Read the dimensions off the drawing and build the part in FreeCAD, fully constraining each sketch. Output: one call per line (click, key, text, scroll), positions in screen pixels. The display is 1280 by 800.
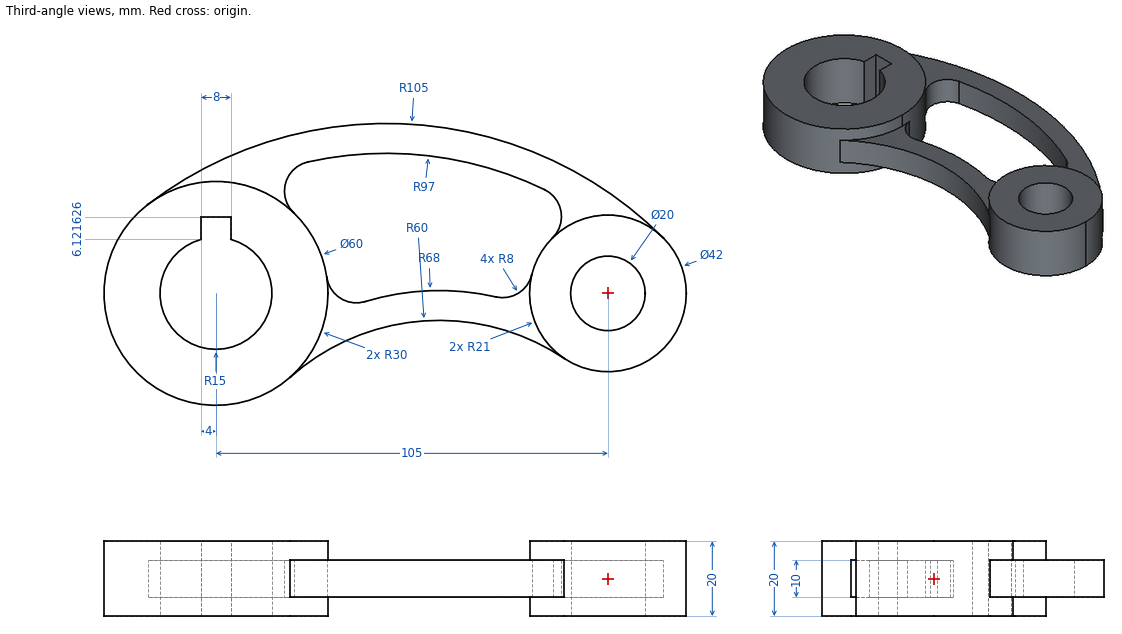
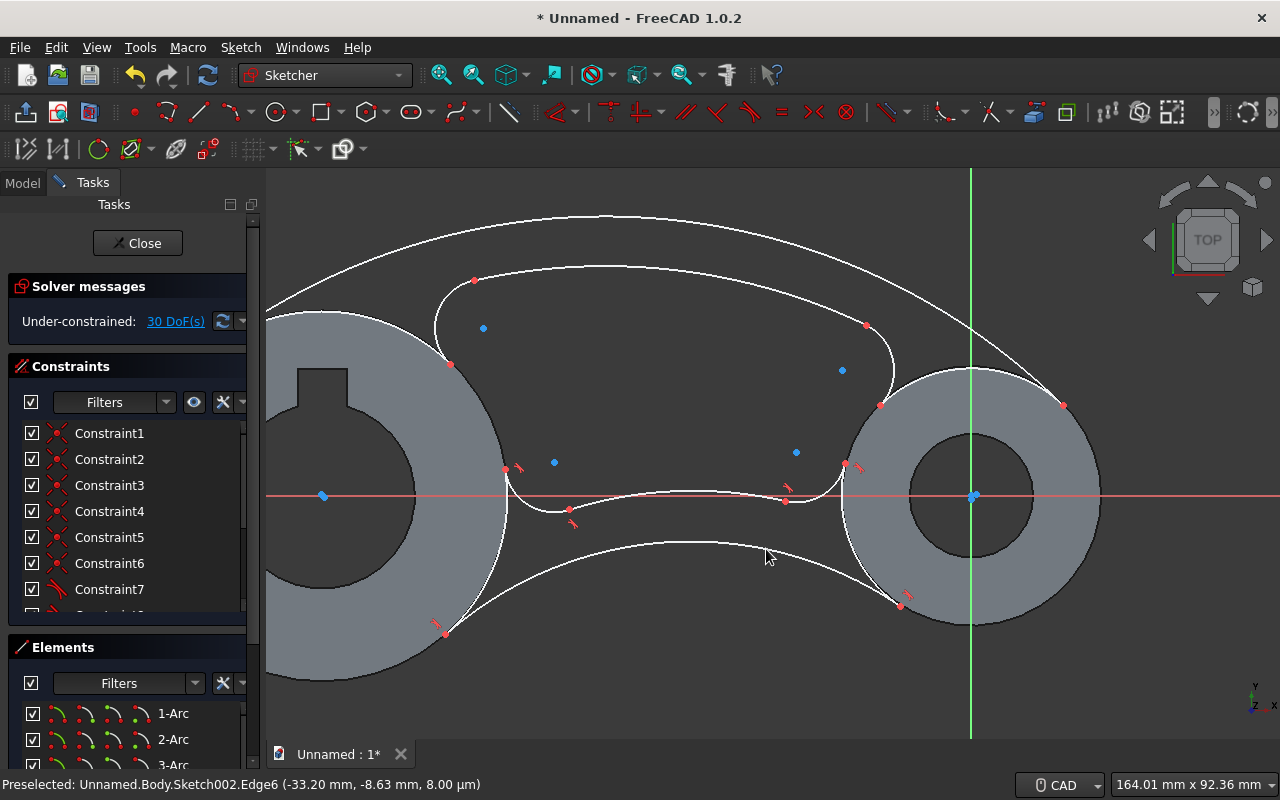
click(829, 256)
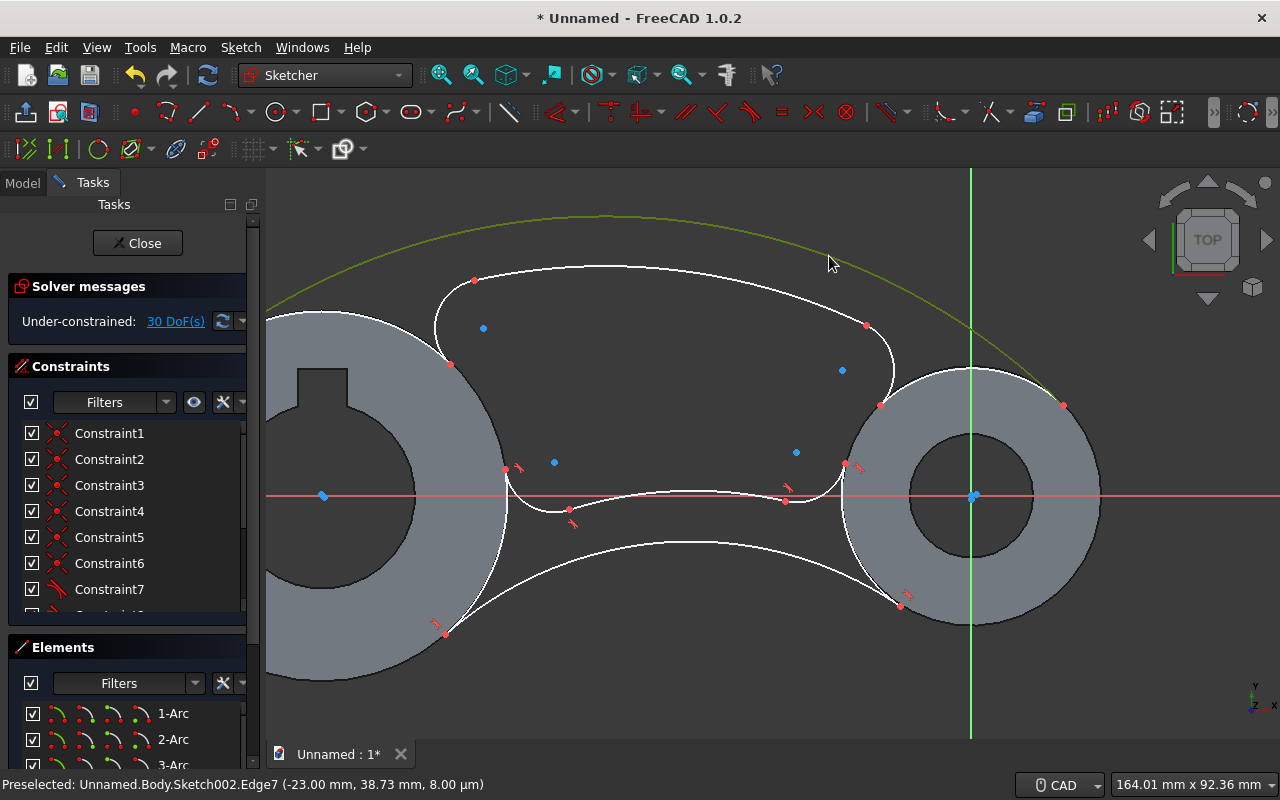
click(384, 322)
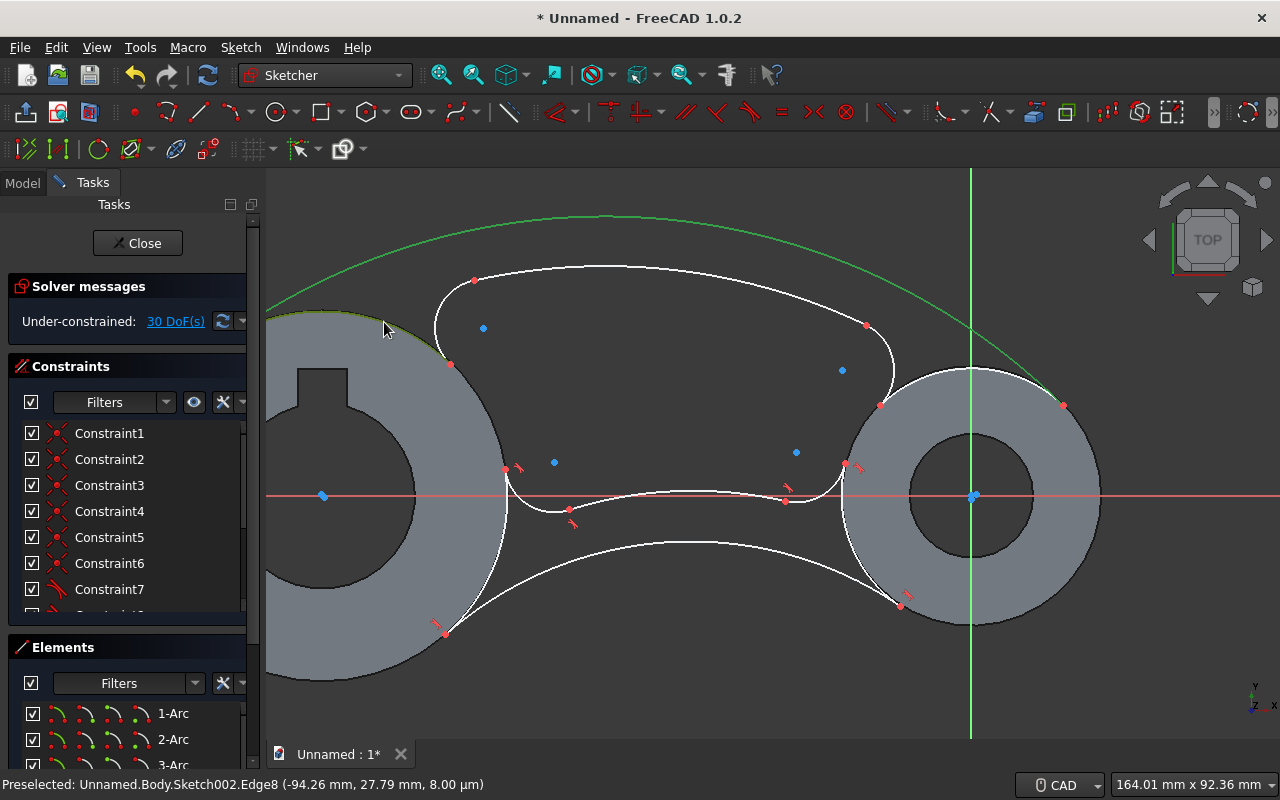
key(t)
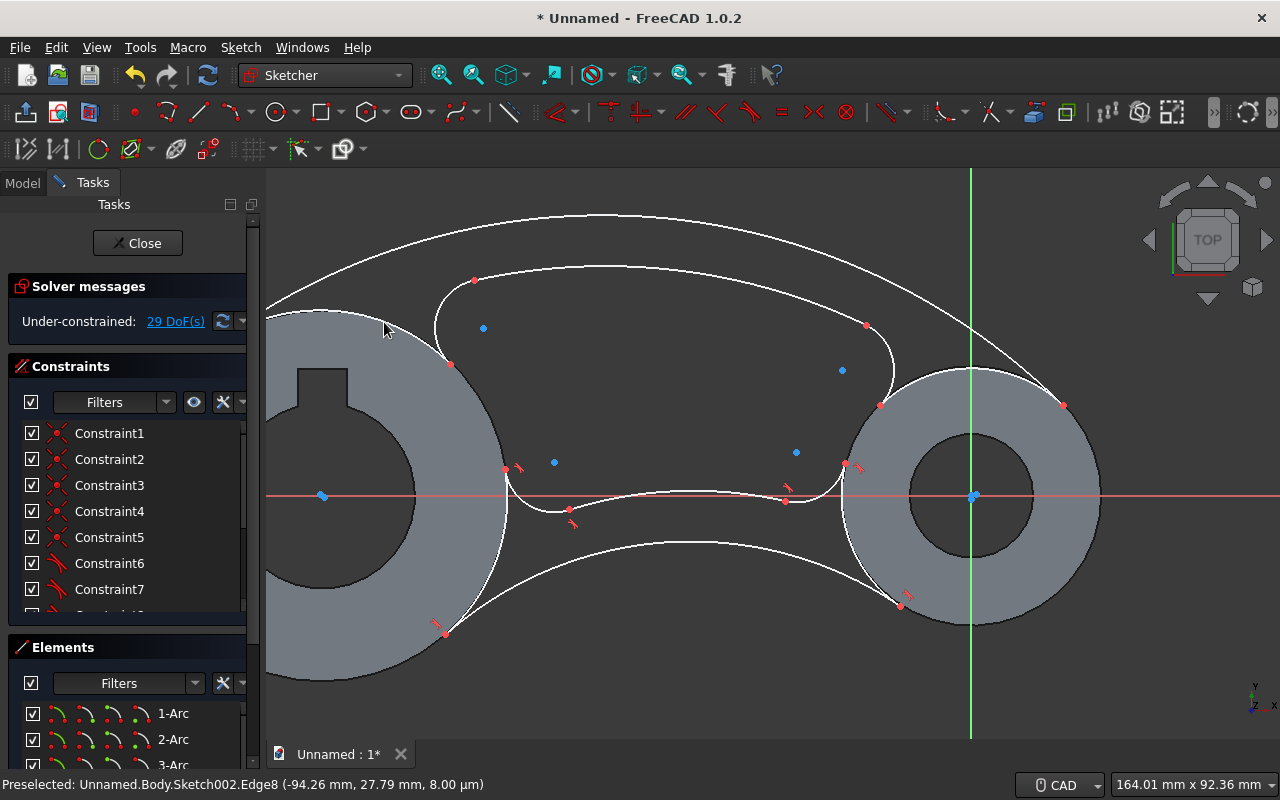
click(829, 256)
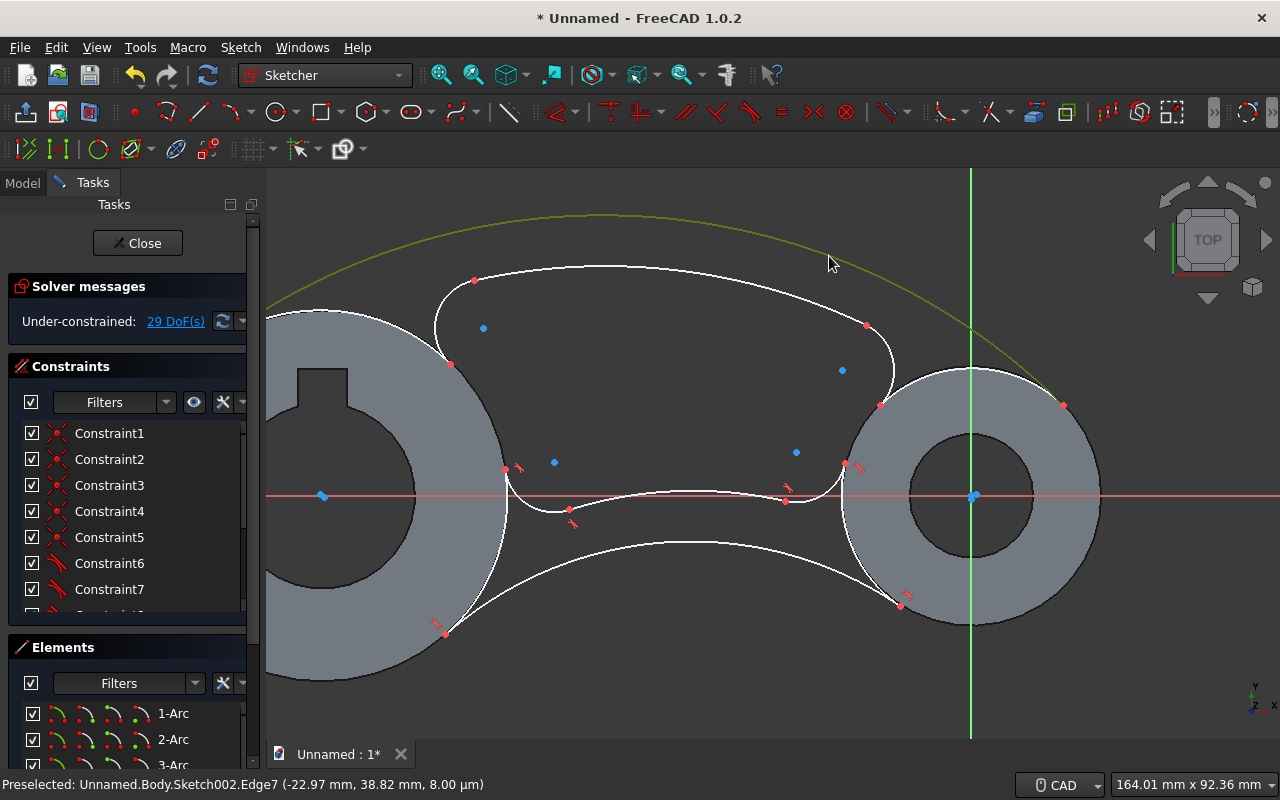
click(1012, 375)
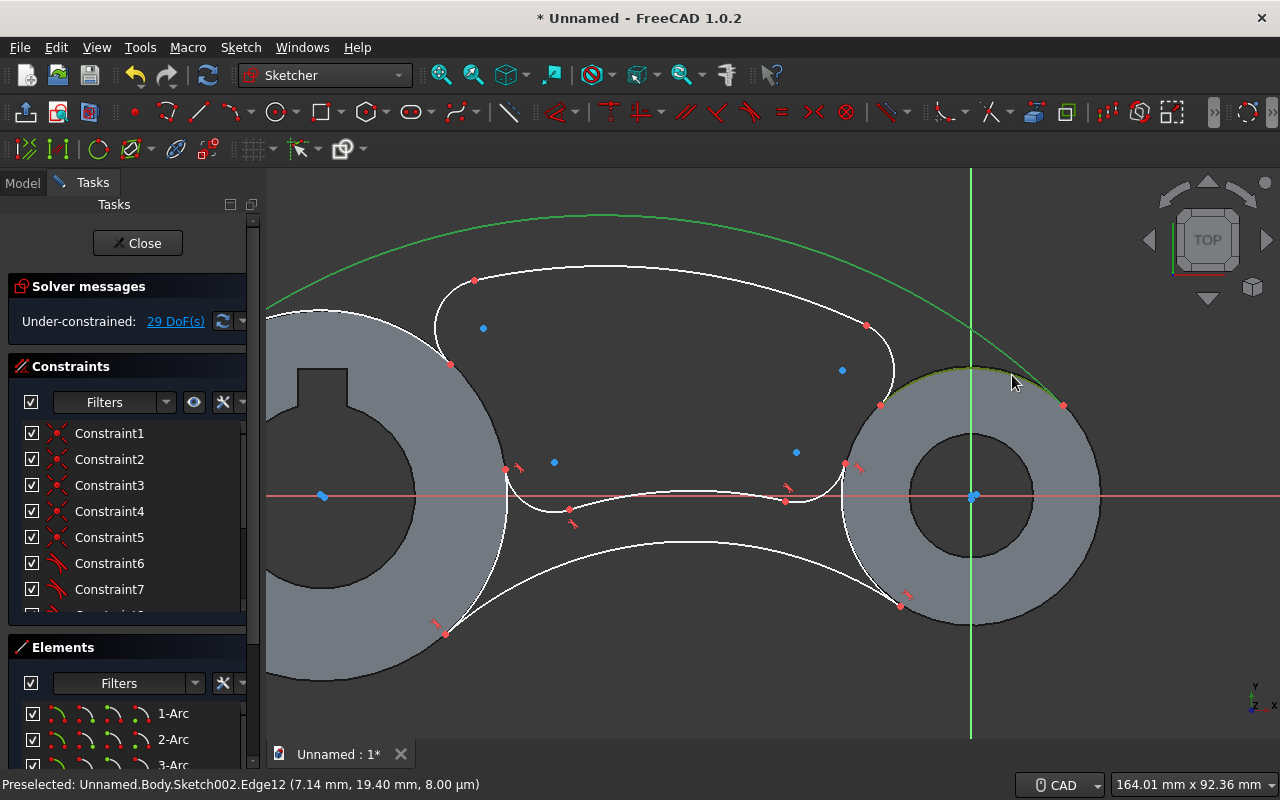
click(750, 112)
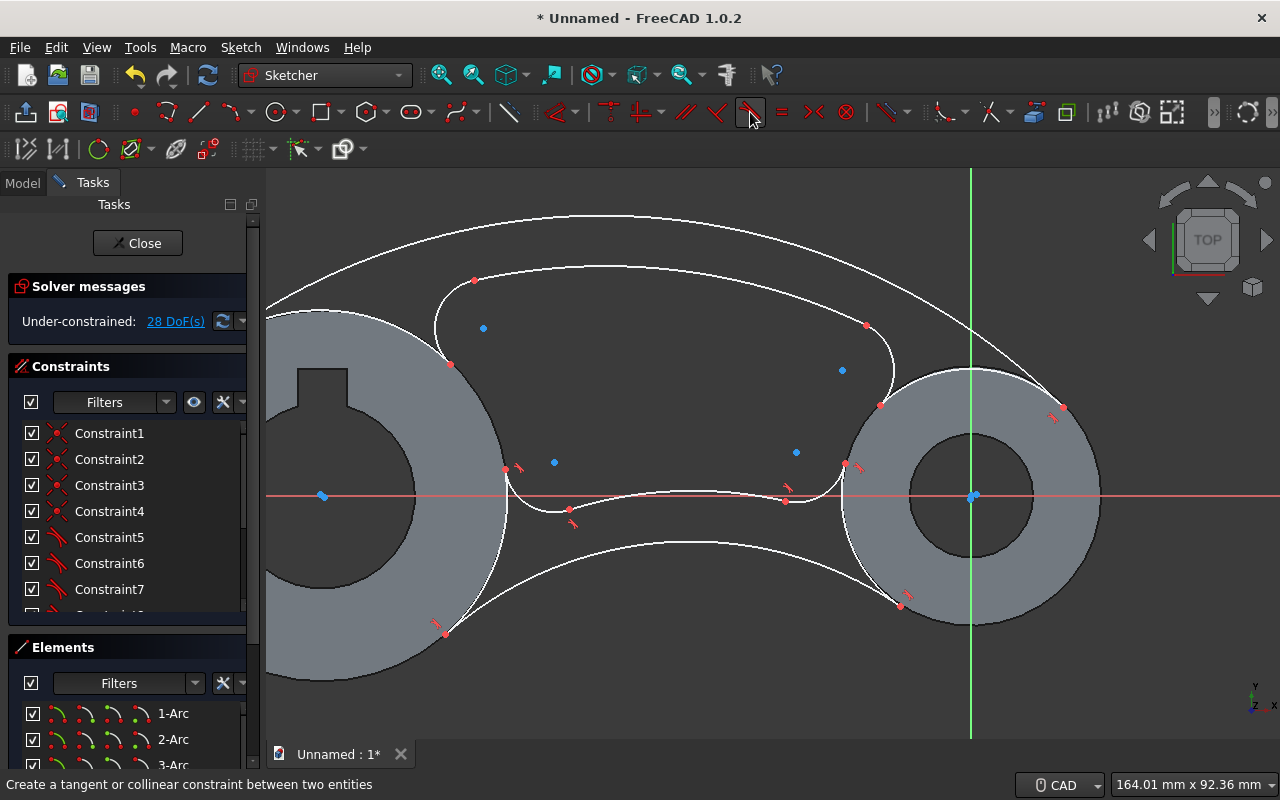
click(384, 322)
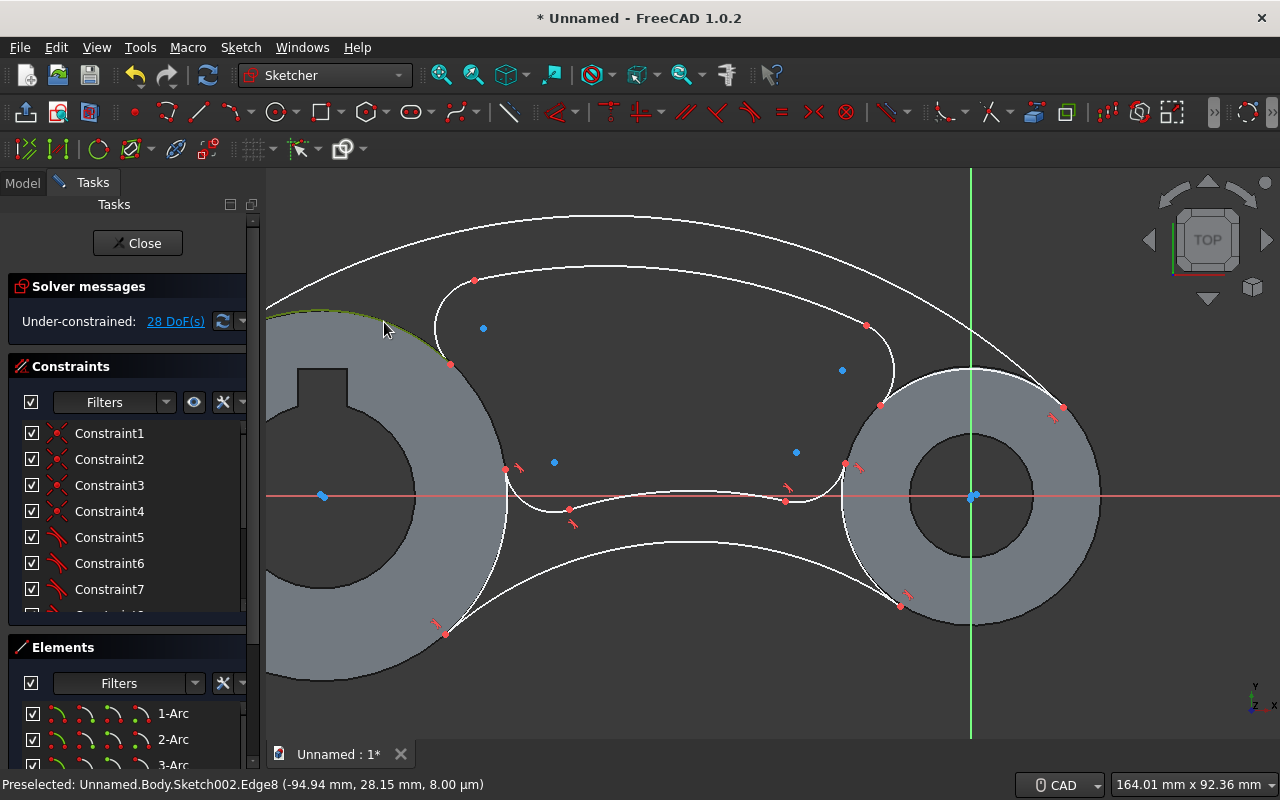
click(447, 296)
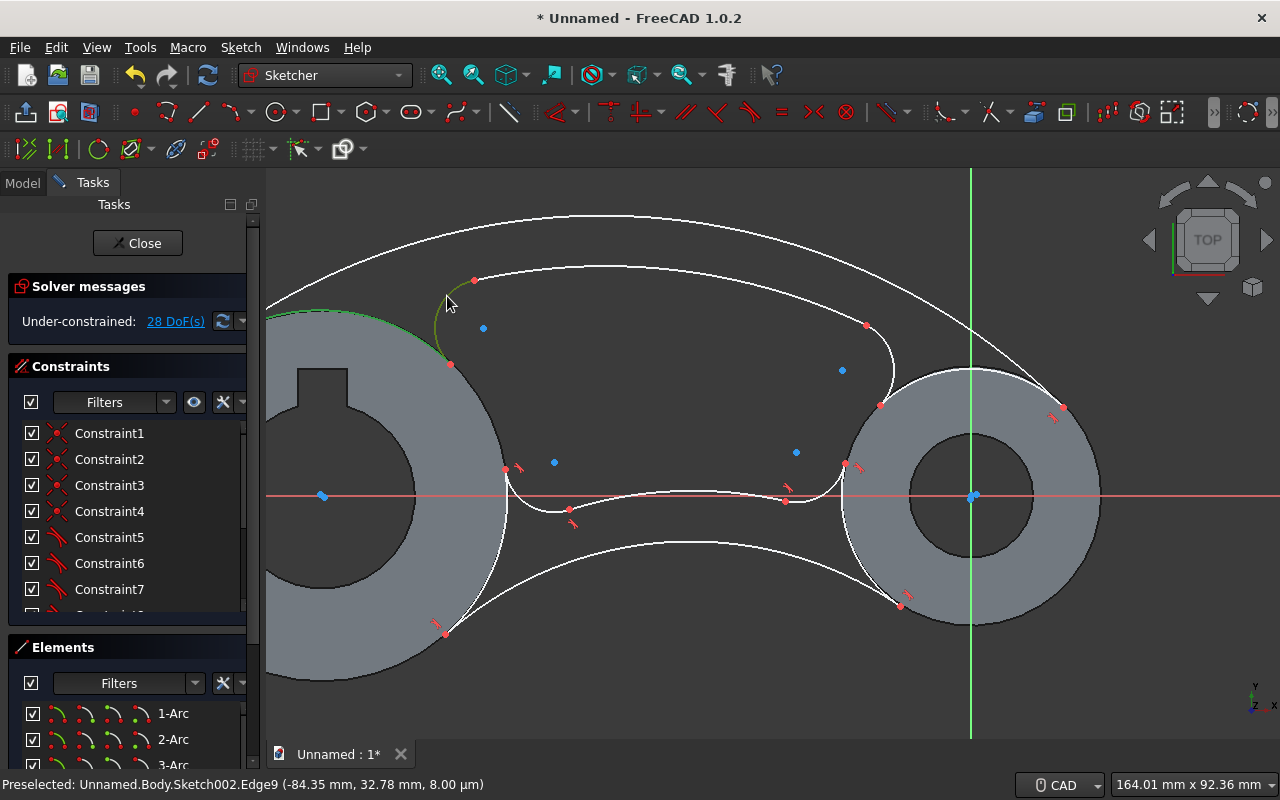
key(t)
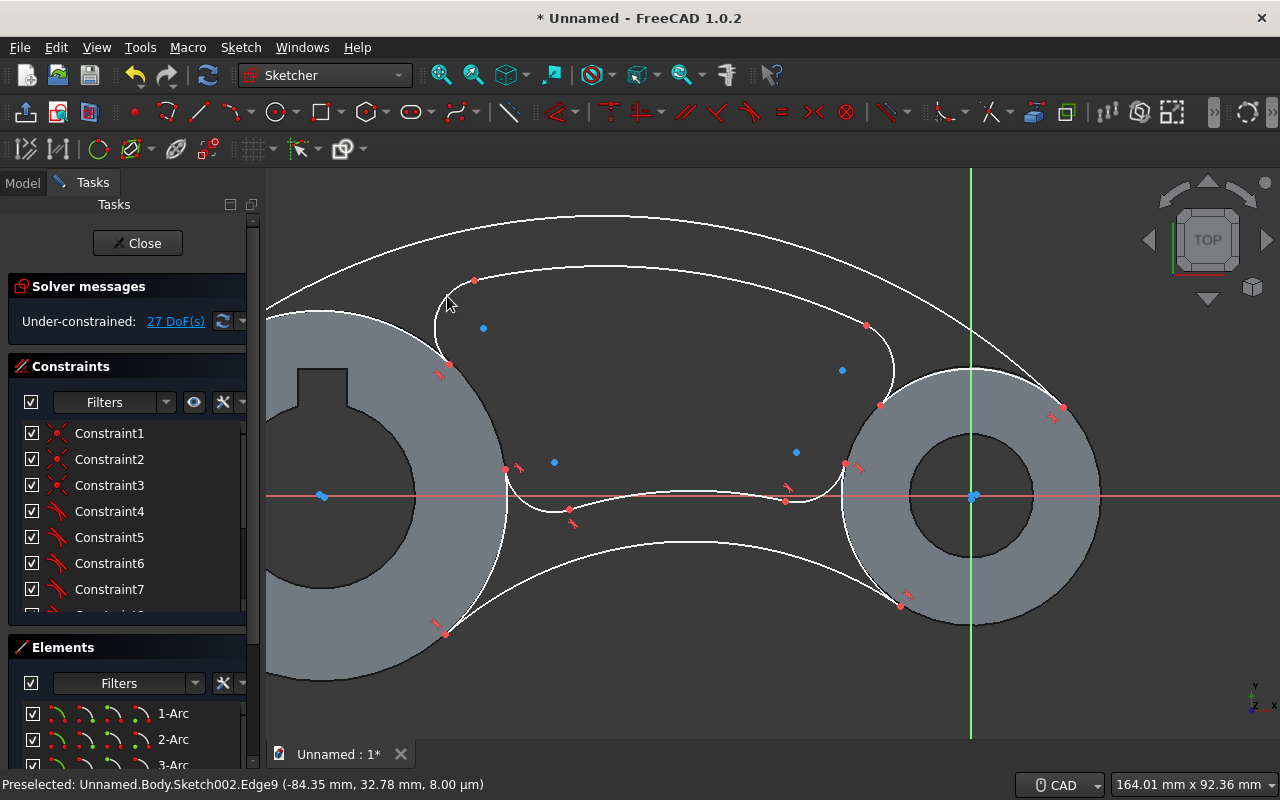
click(447, 296)